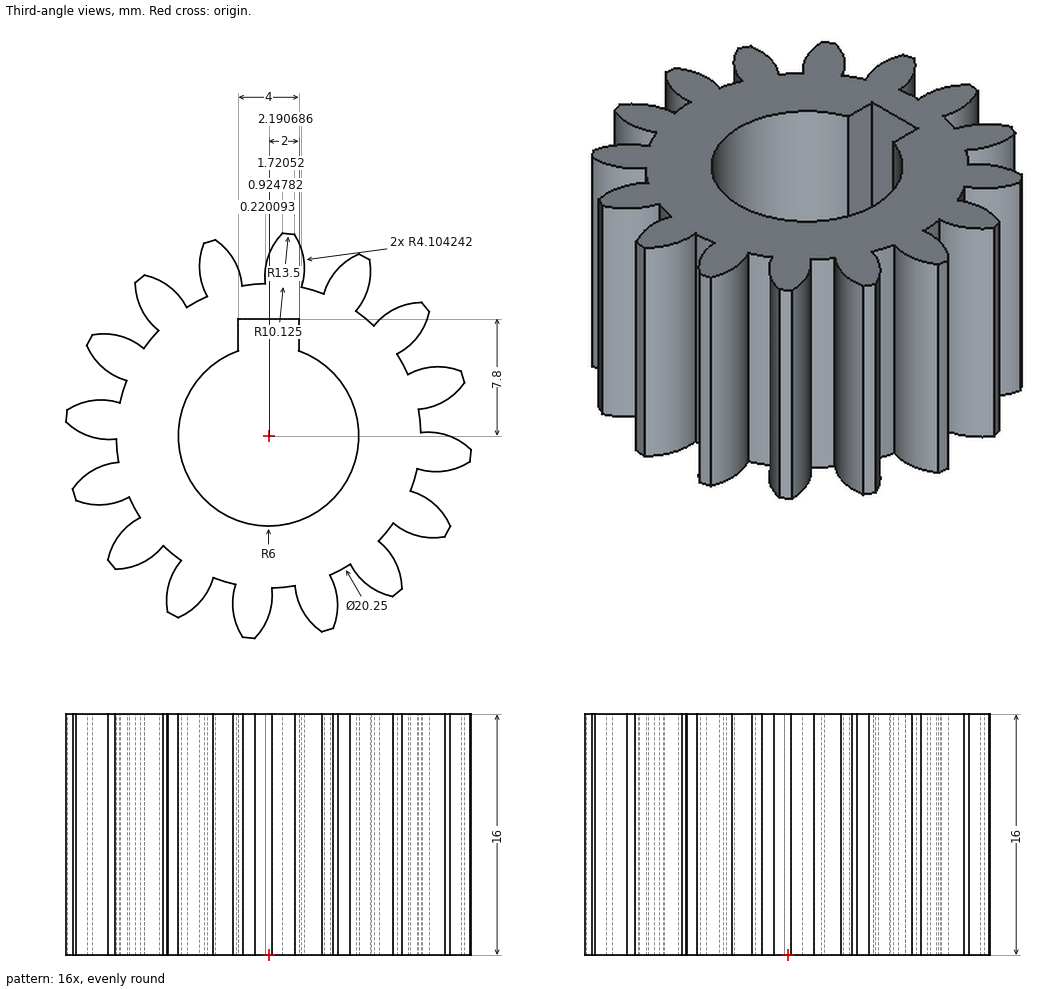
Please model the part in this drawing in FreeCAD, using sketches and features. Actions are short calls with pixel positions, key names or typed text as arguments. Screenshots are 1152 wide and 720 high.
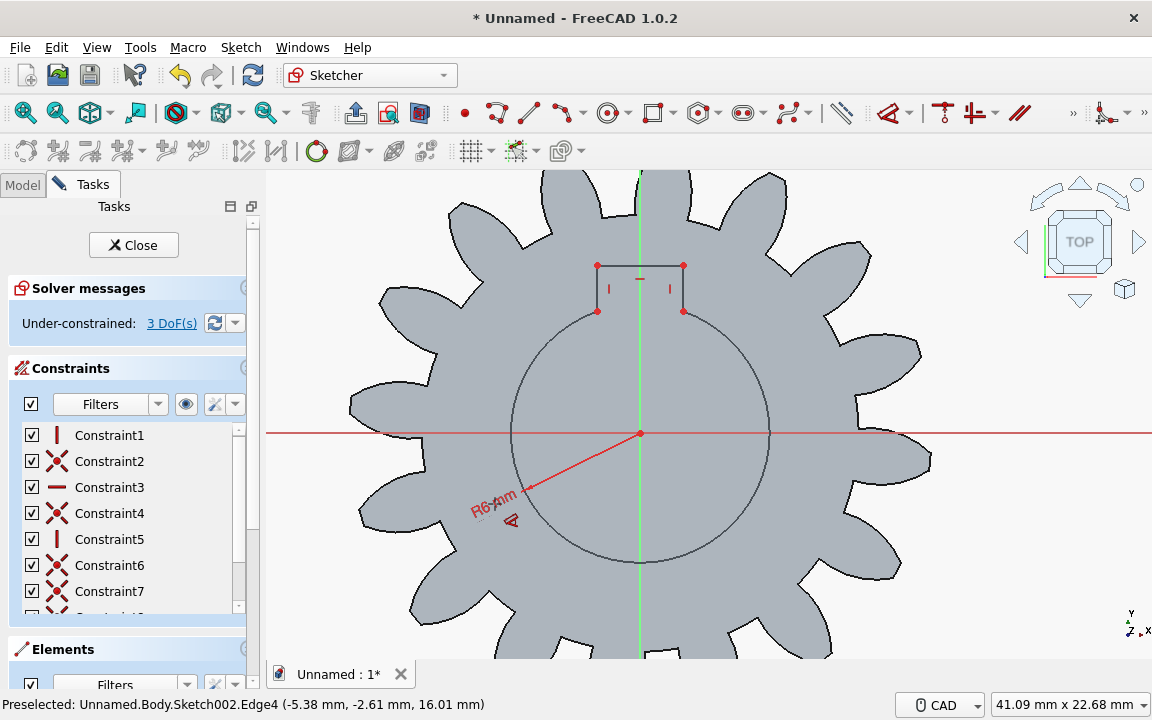
click(657, 266)
click(620, 232)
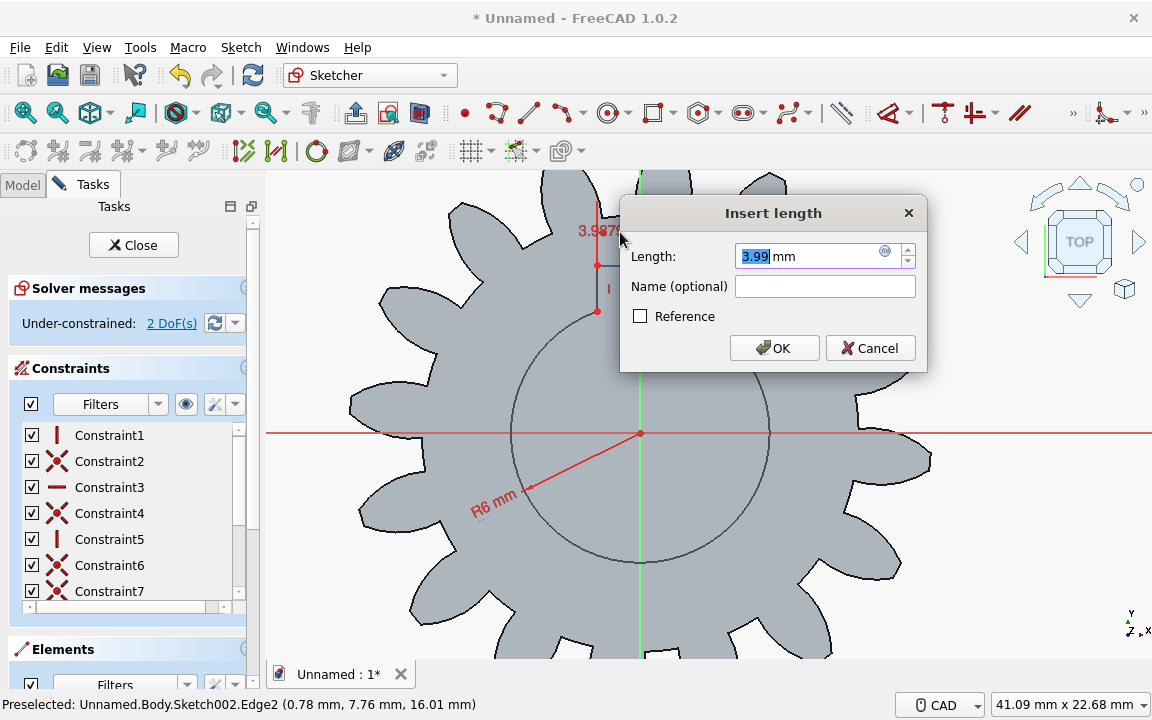
text(4)
key(Return)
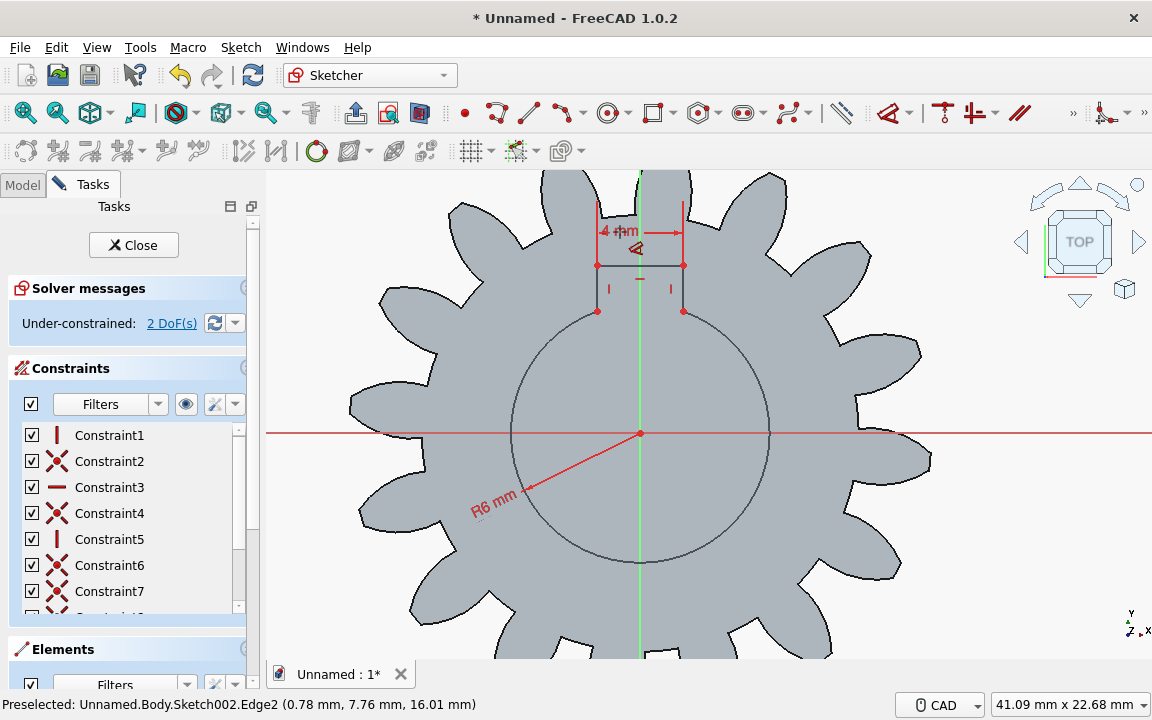
click(683, 311)
click(662, 467)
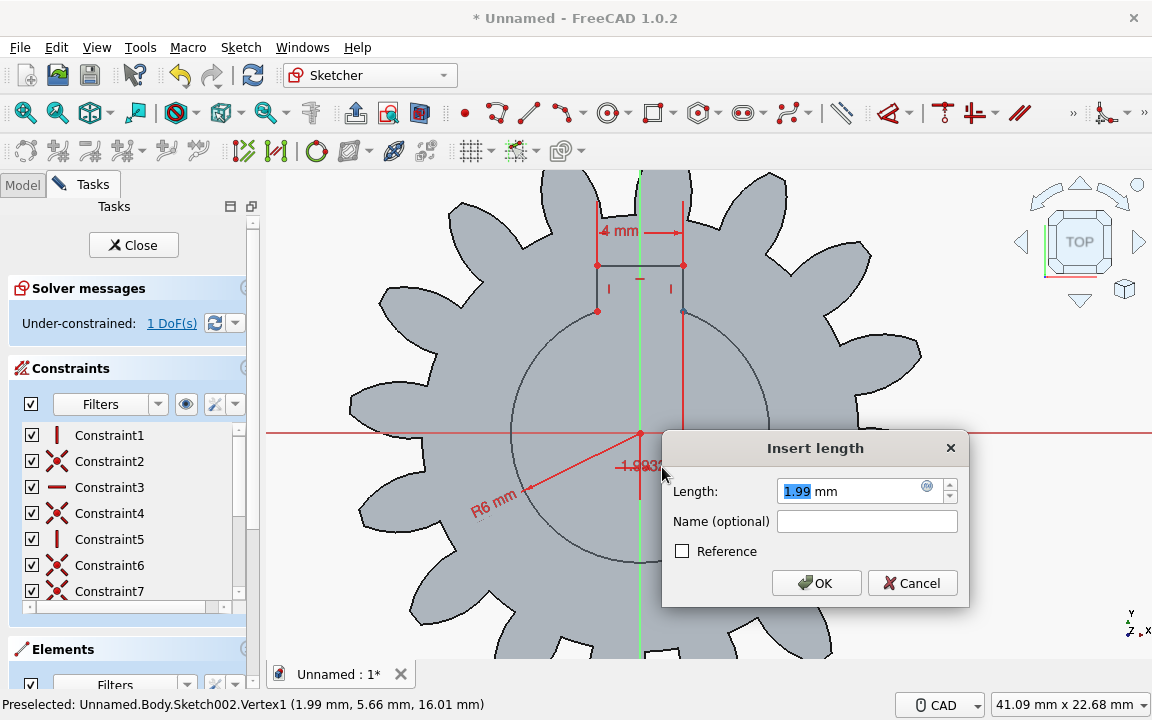
text(2)
key(Return)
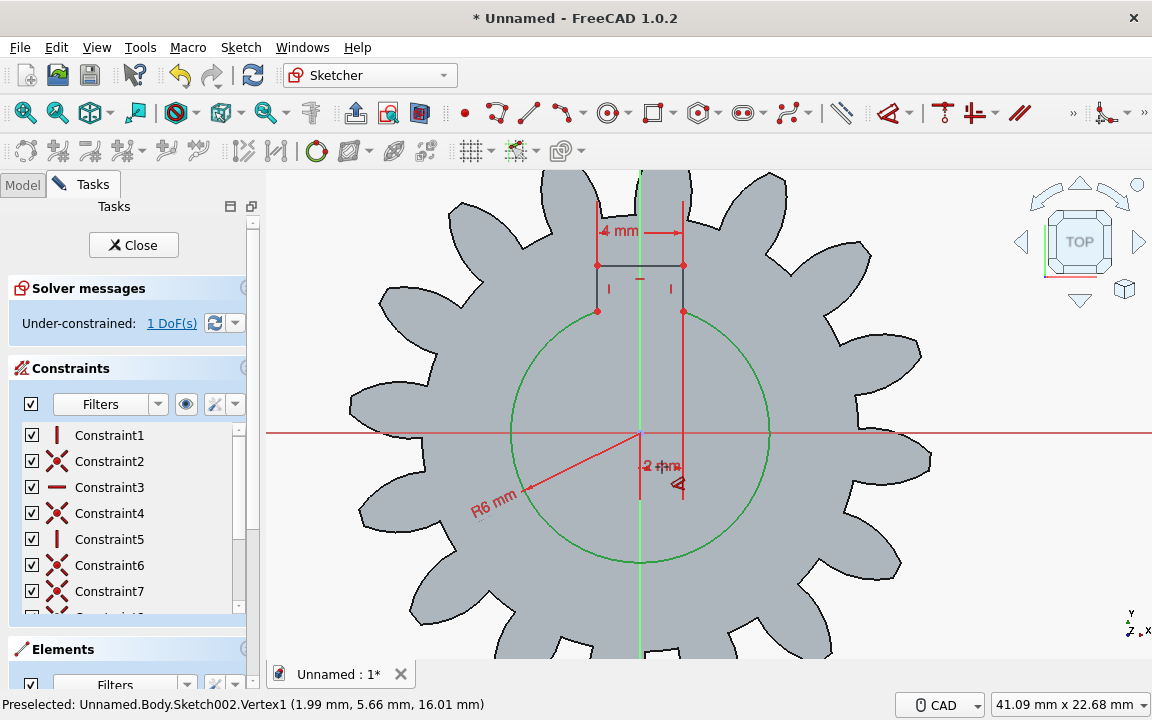
click(683, 266)
click(717, 350)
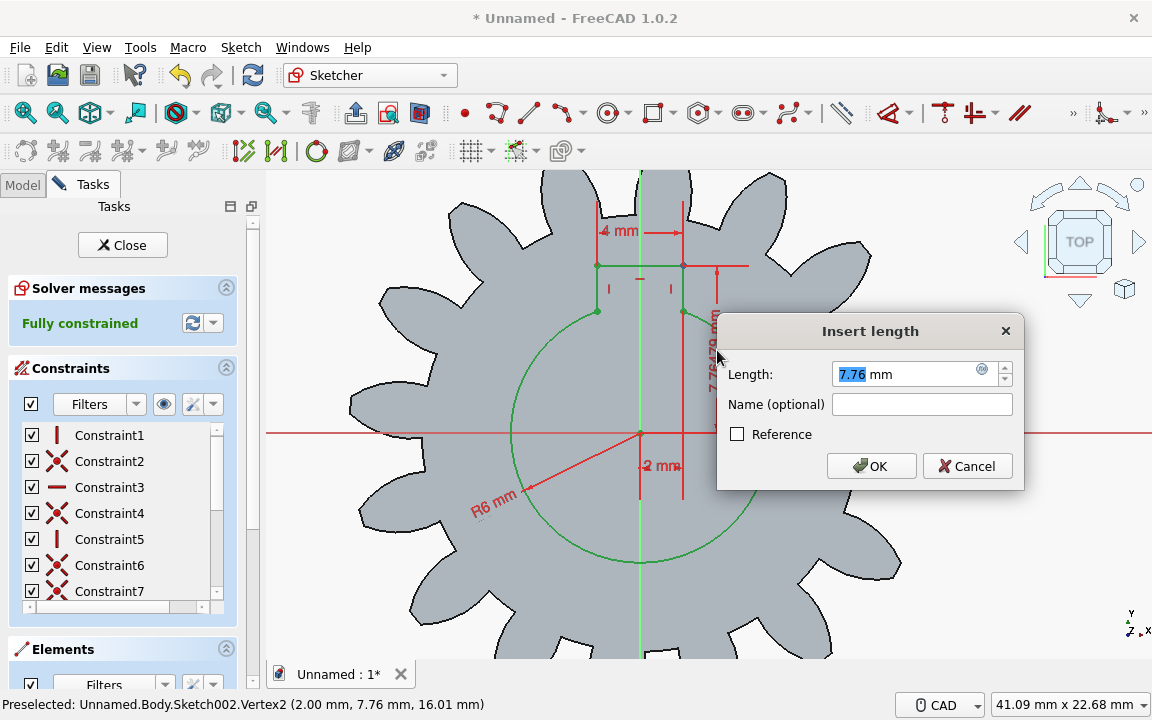
text(7.8)
key(Return)
key(Escape)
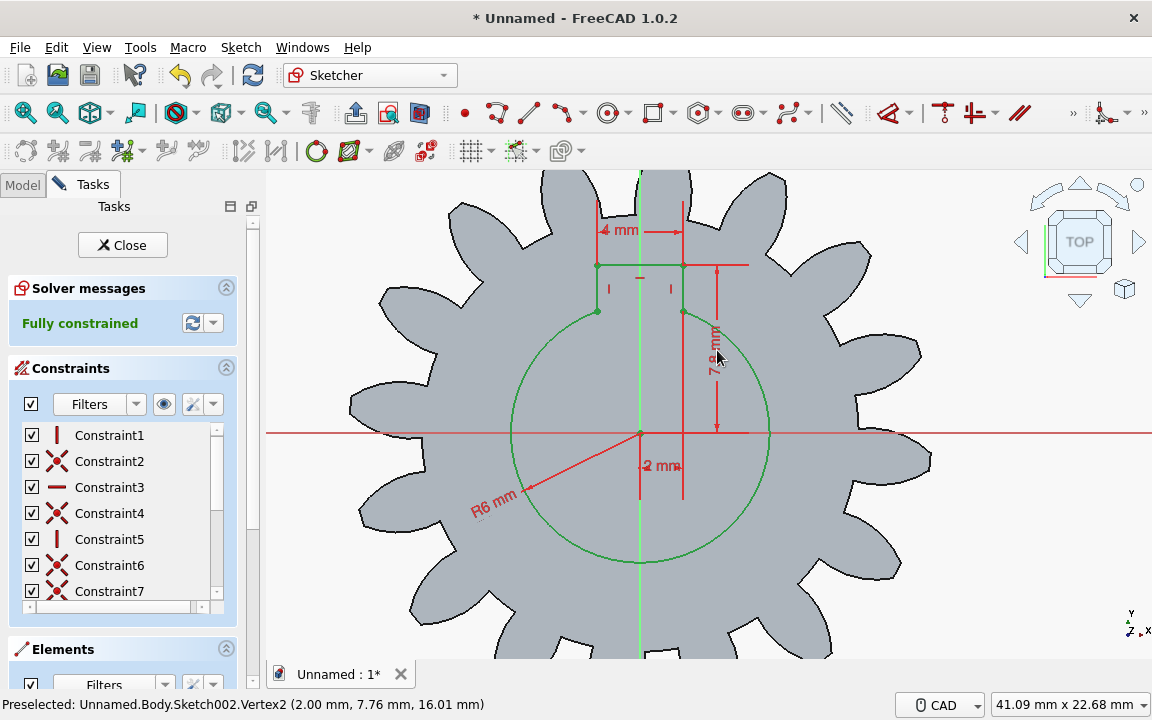
click(123, 245)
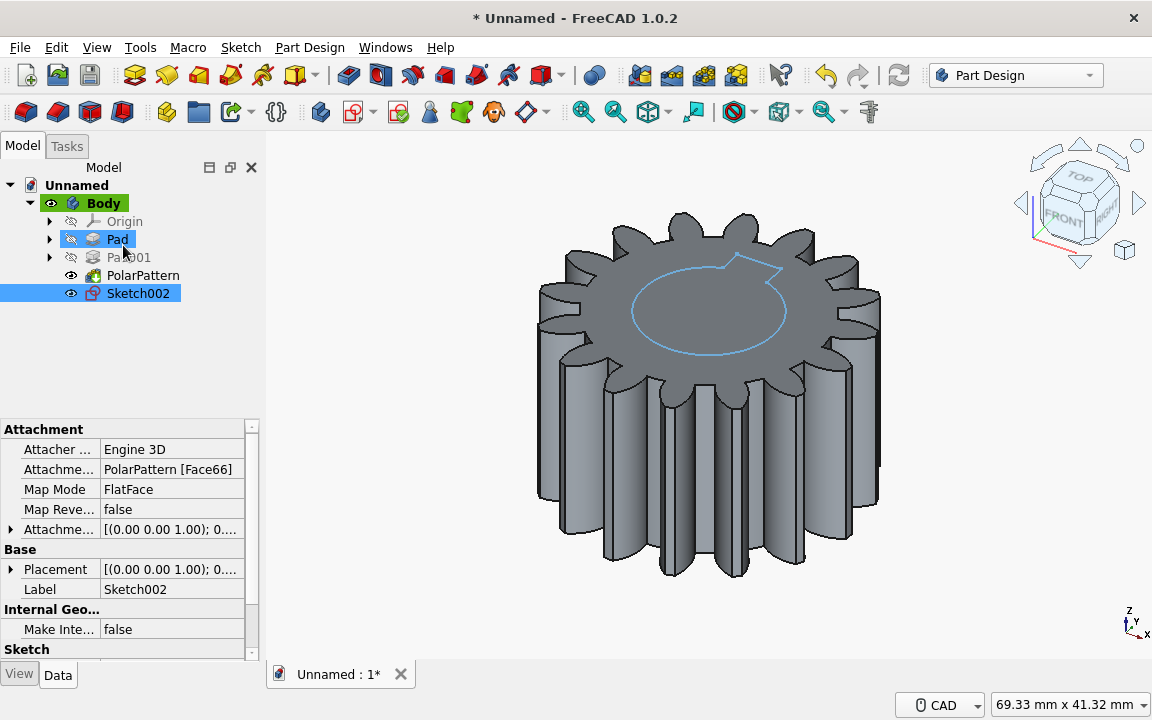
click(350, 76)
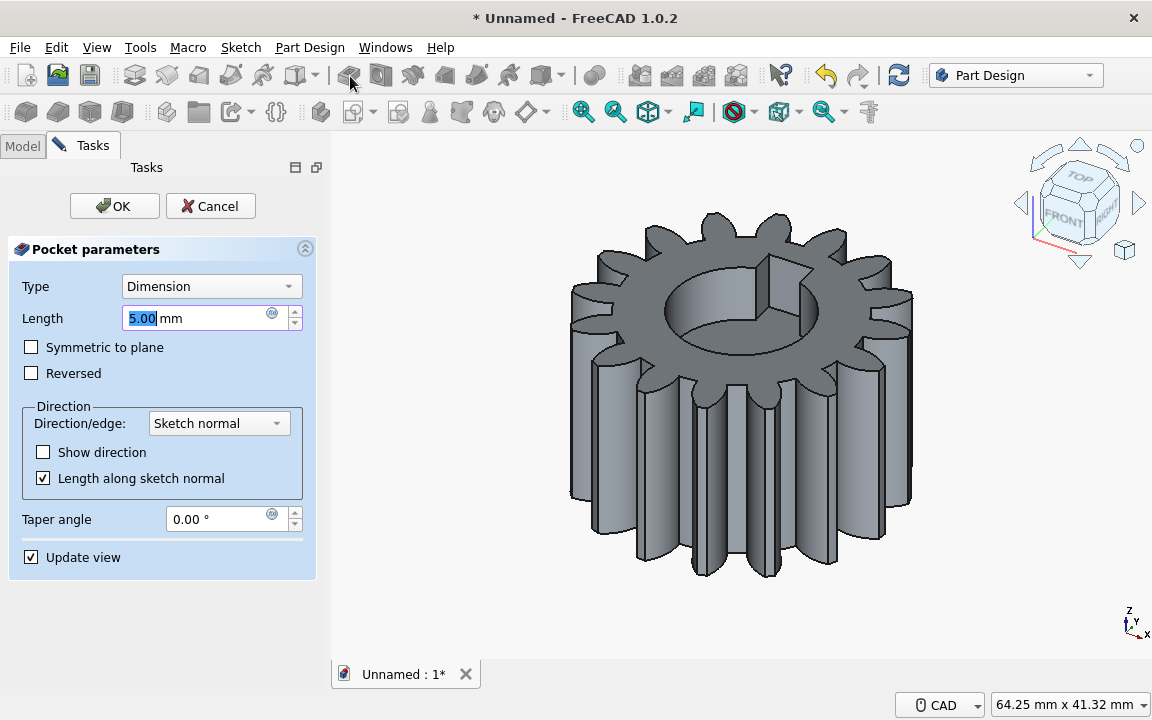
text(16)
key(Tab)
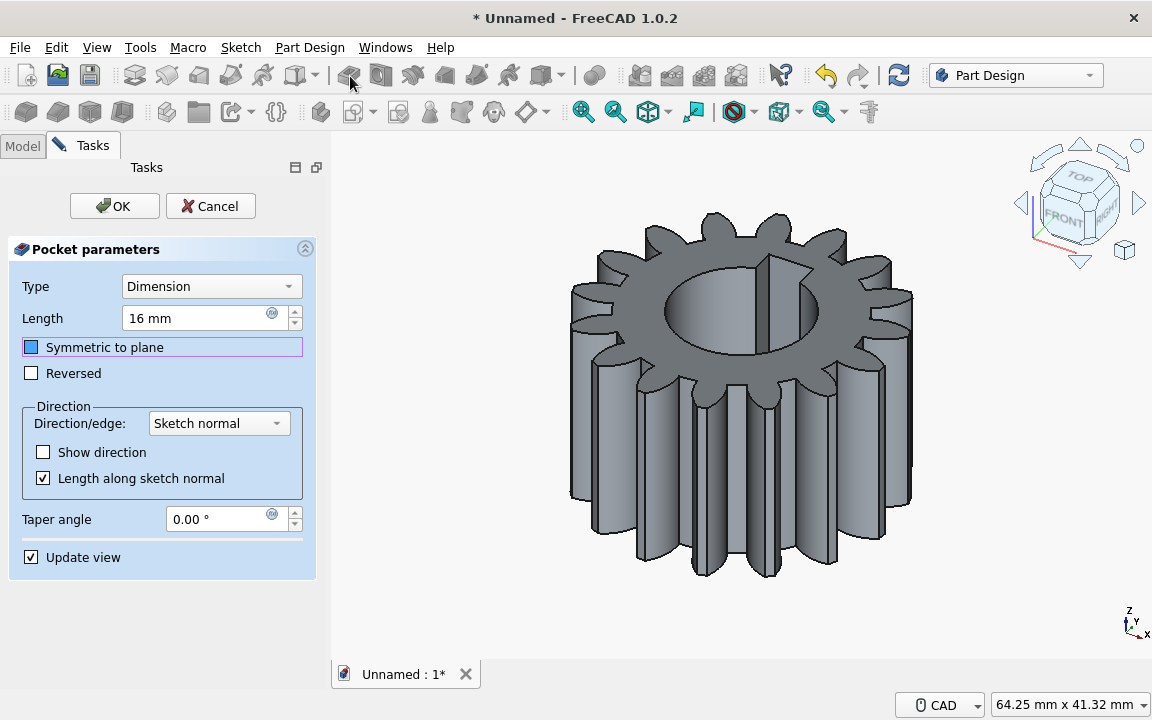
click(115, 206)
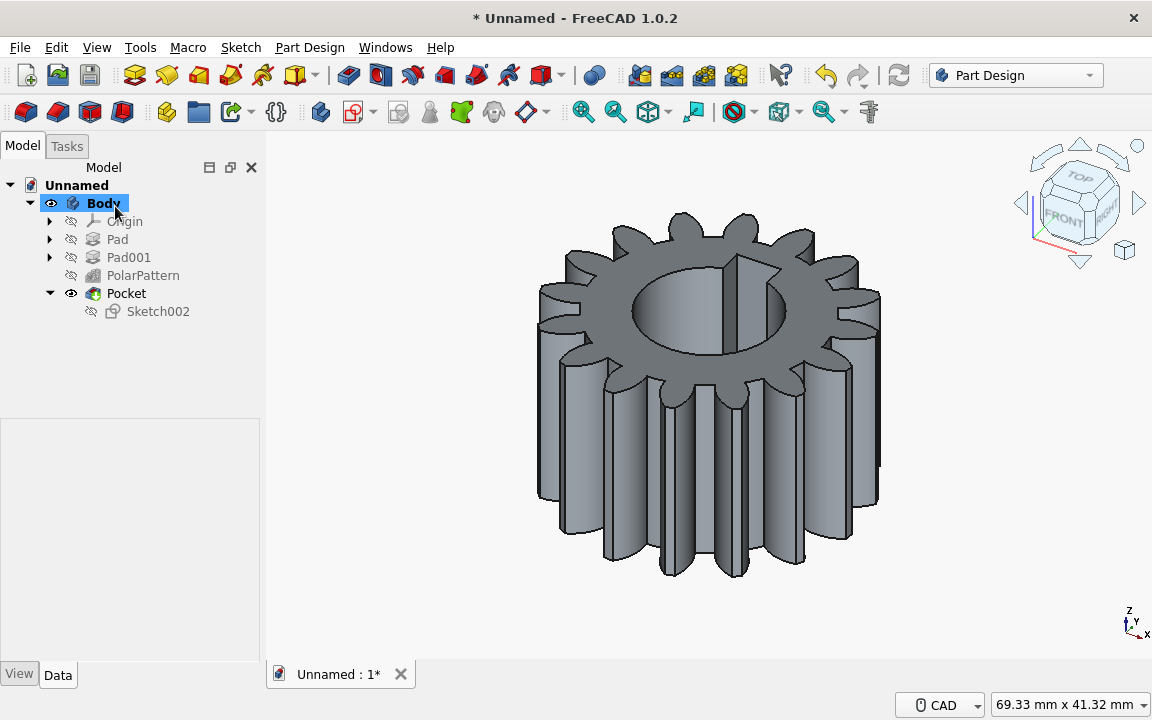
key(0)